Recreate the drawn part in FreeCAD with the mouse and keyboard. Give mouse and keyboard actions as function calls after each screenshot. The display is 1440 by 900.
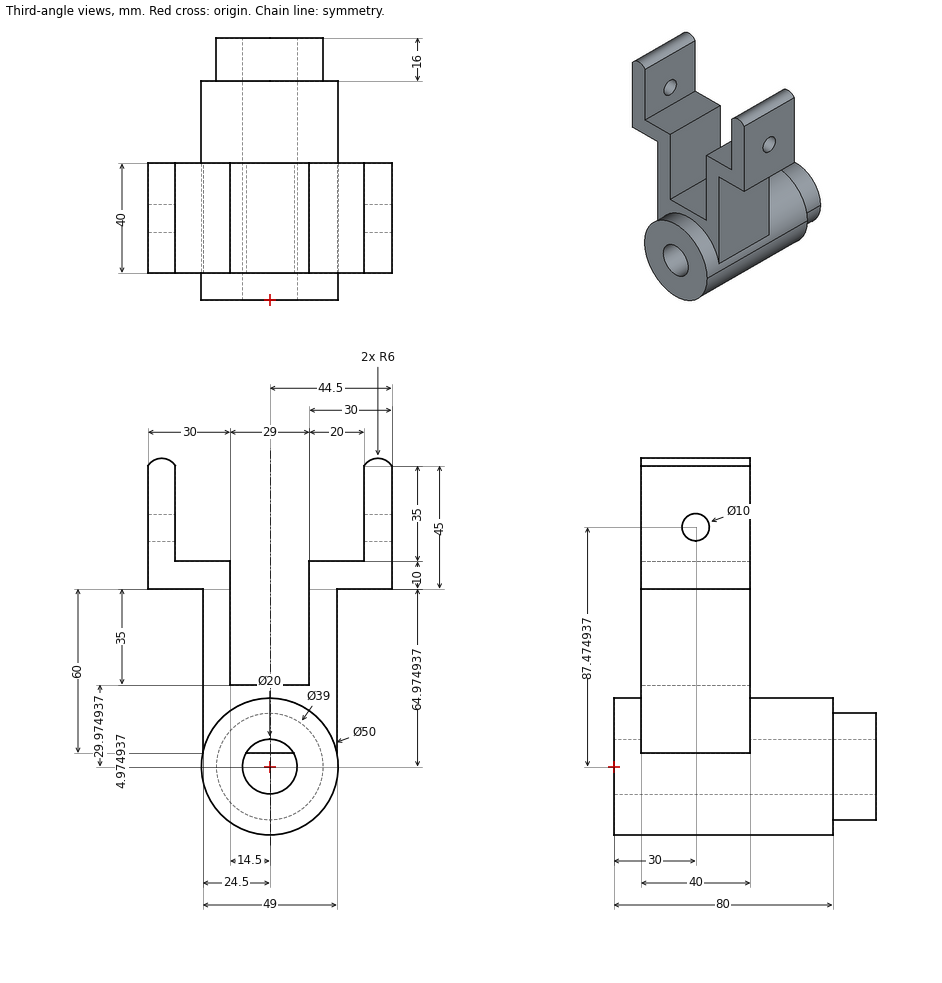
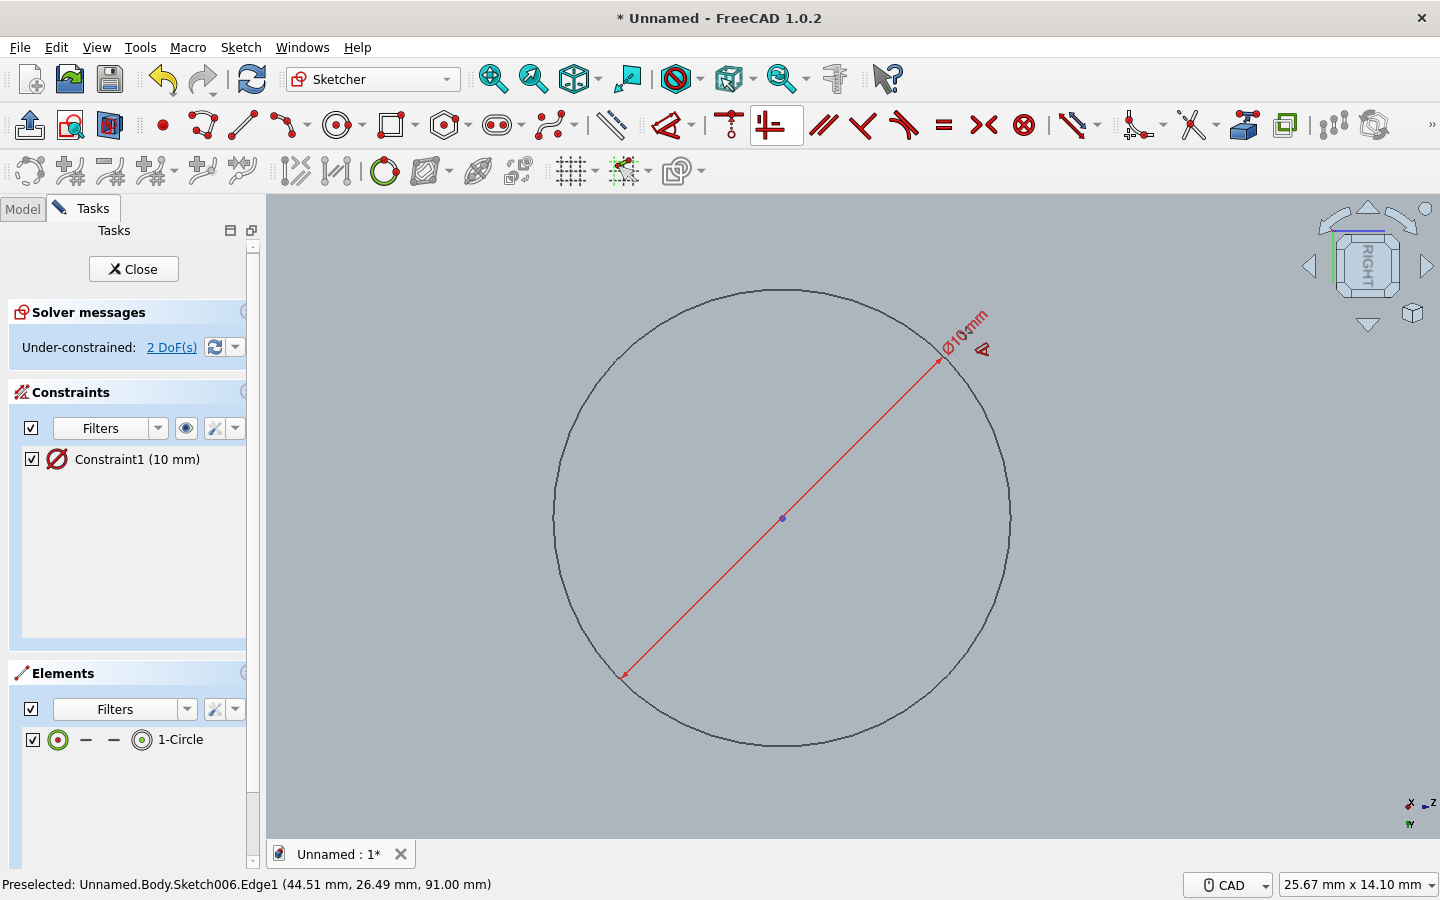
click(782, 518)
click(816, 370)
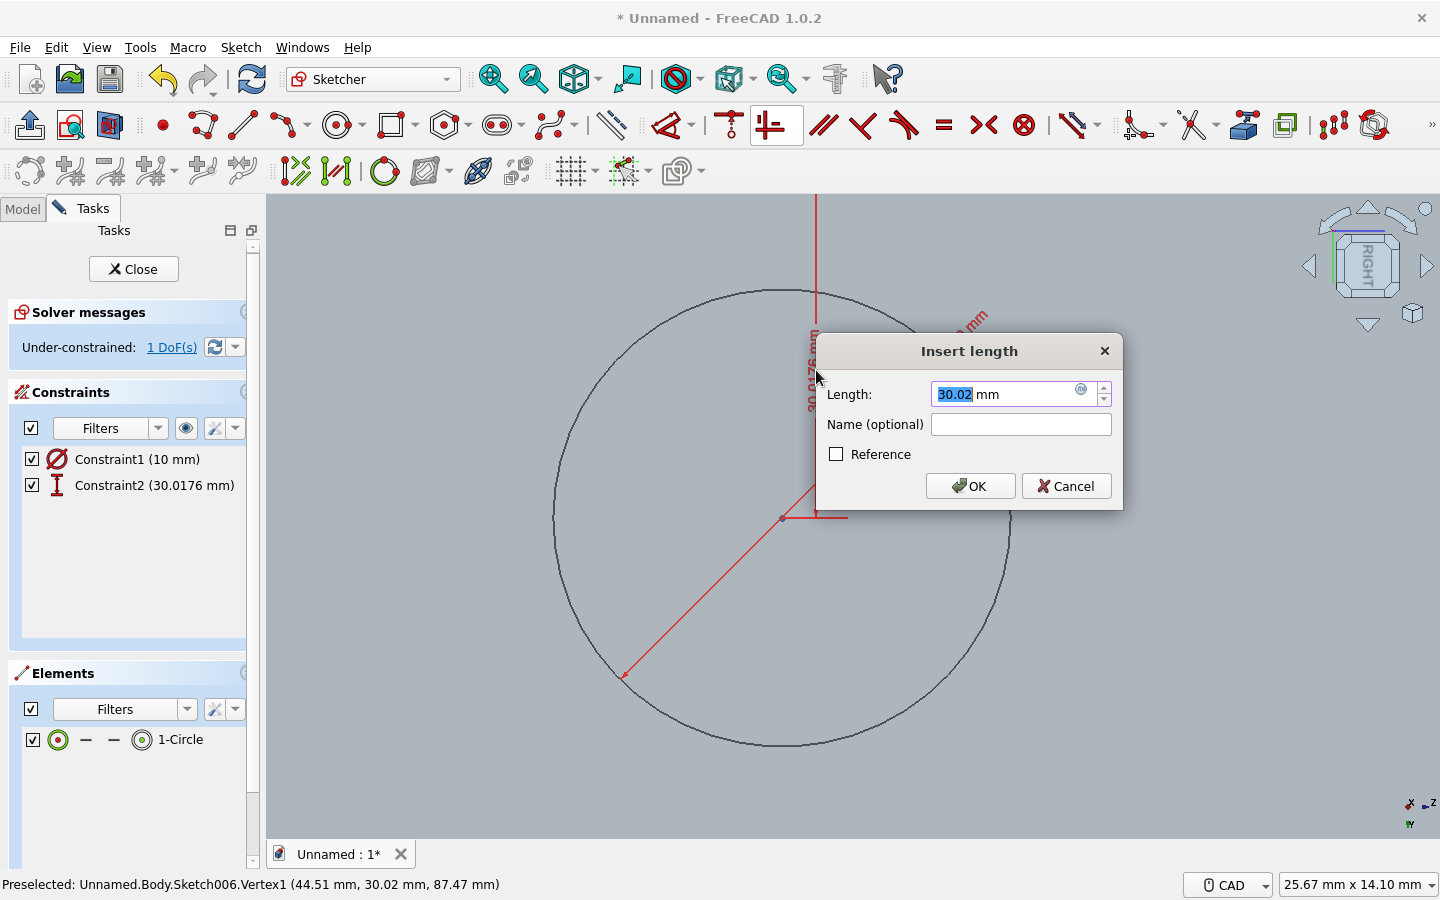
text(30)
key(Return)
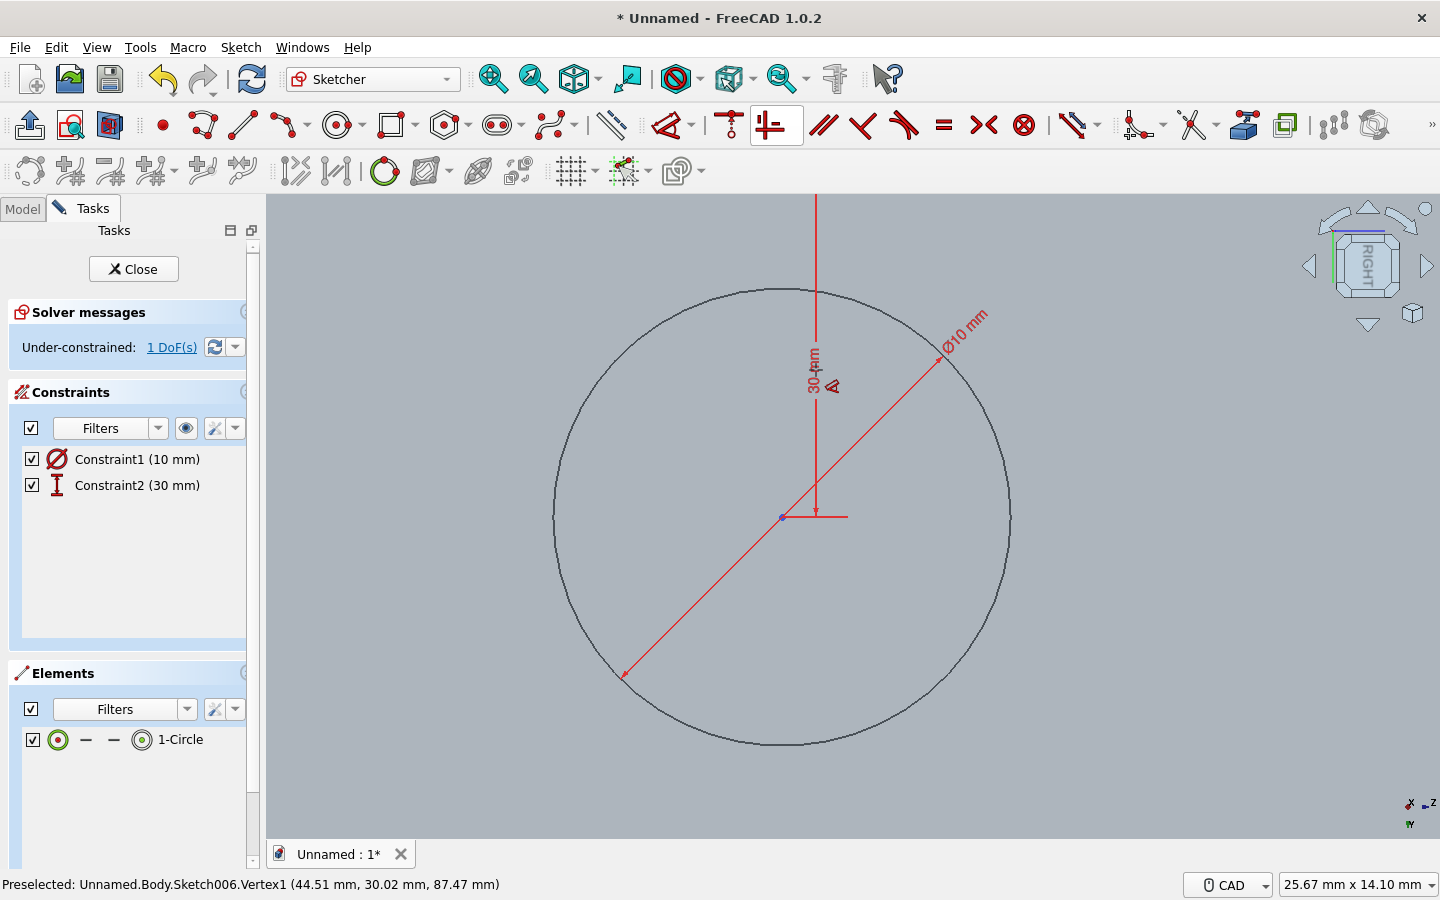
click(782, 517)
click(538, 551)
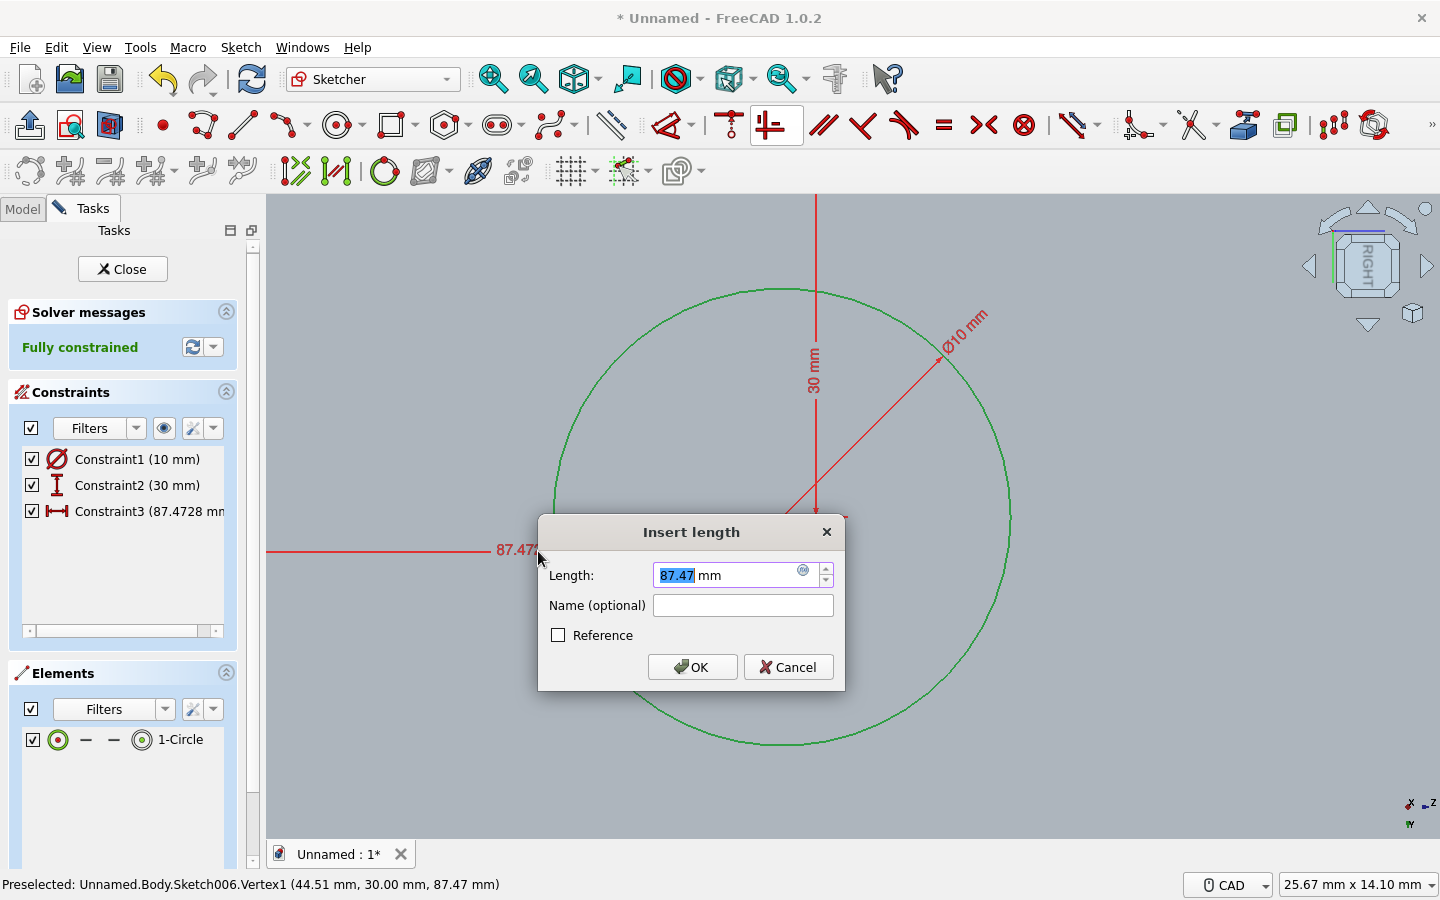
text(87.474937)
key(Return)
key(Escape)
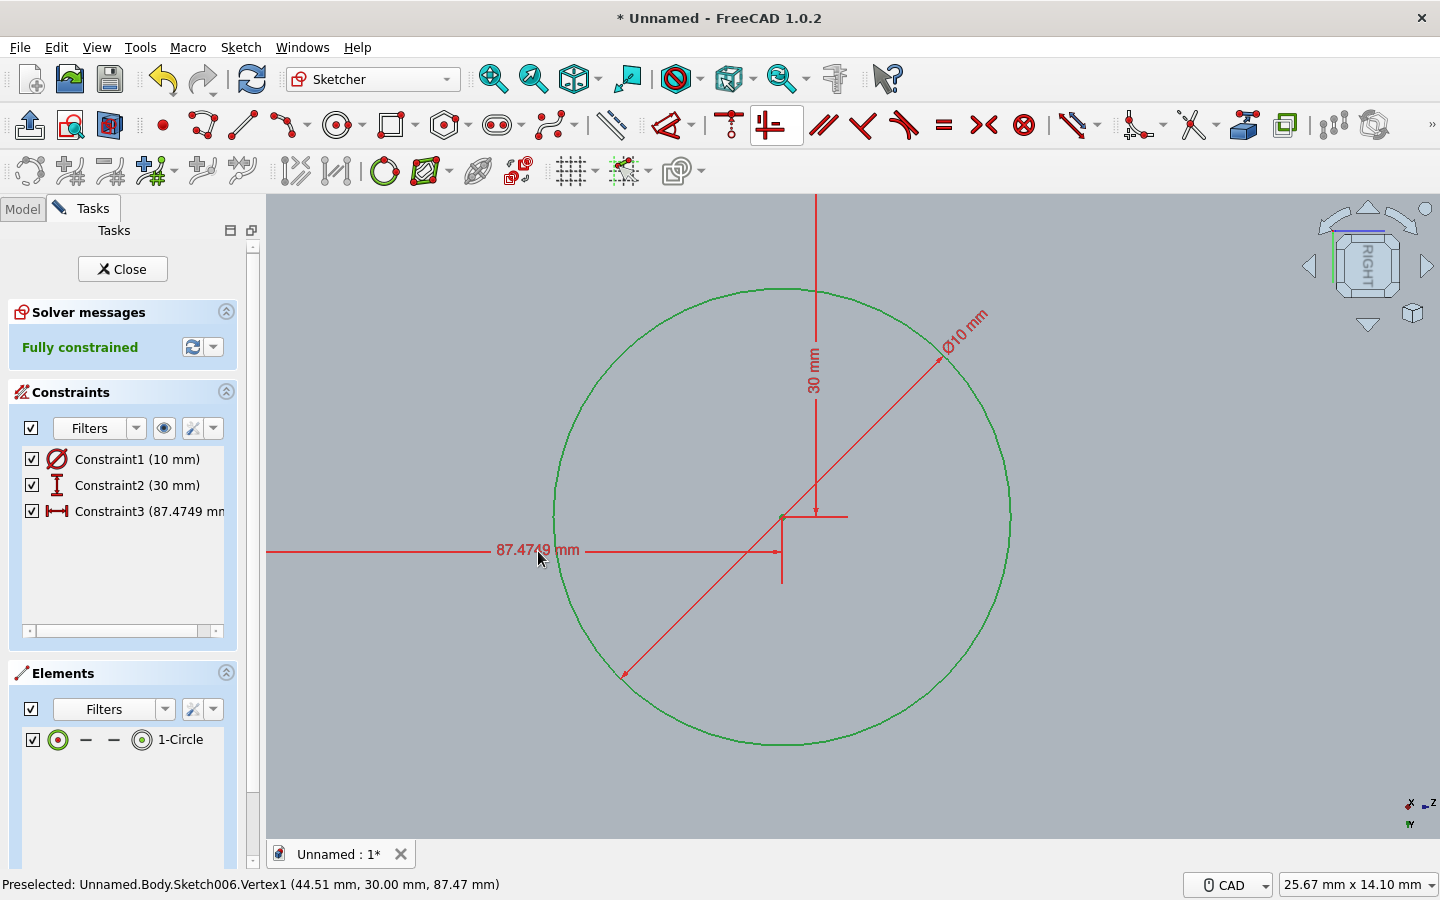
click(123, 269)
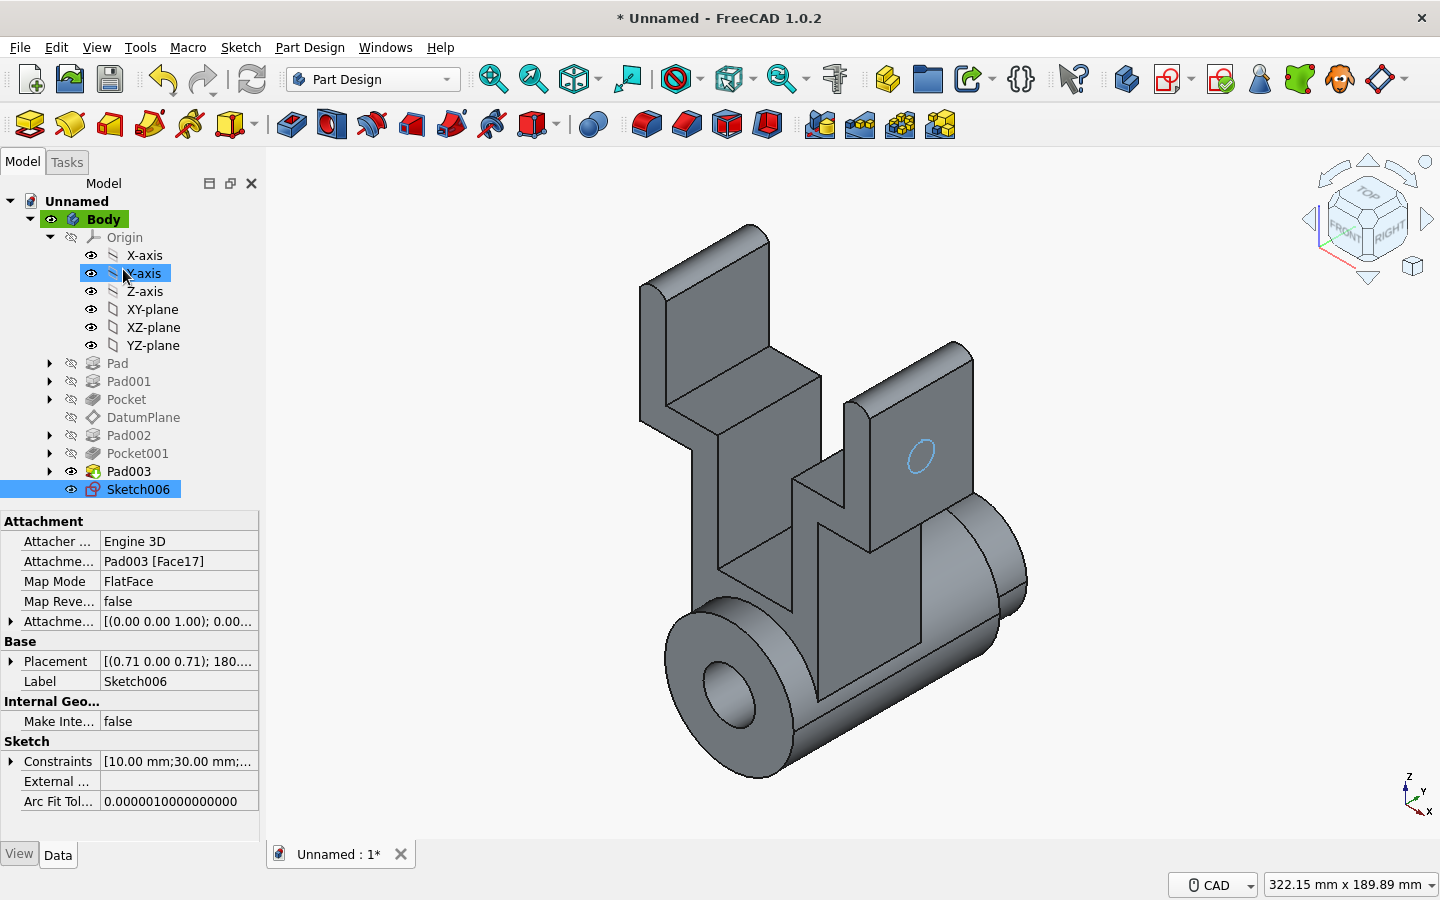
click(292, 124)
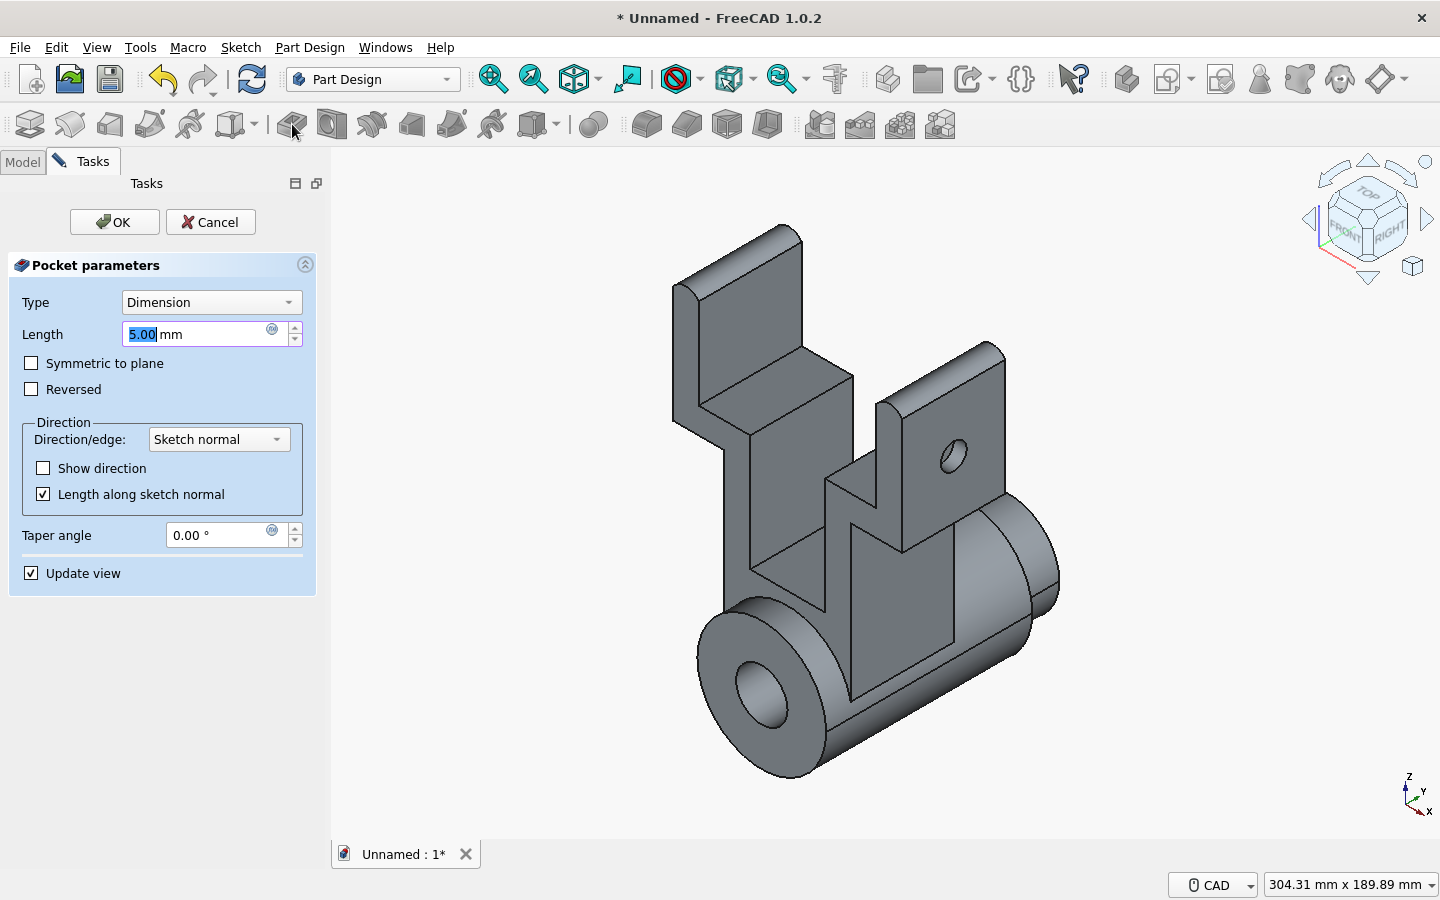
click(212, 302)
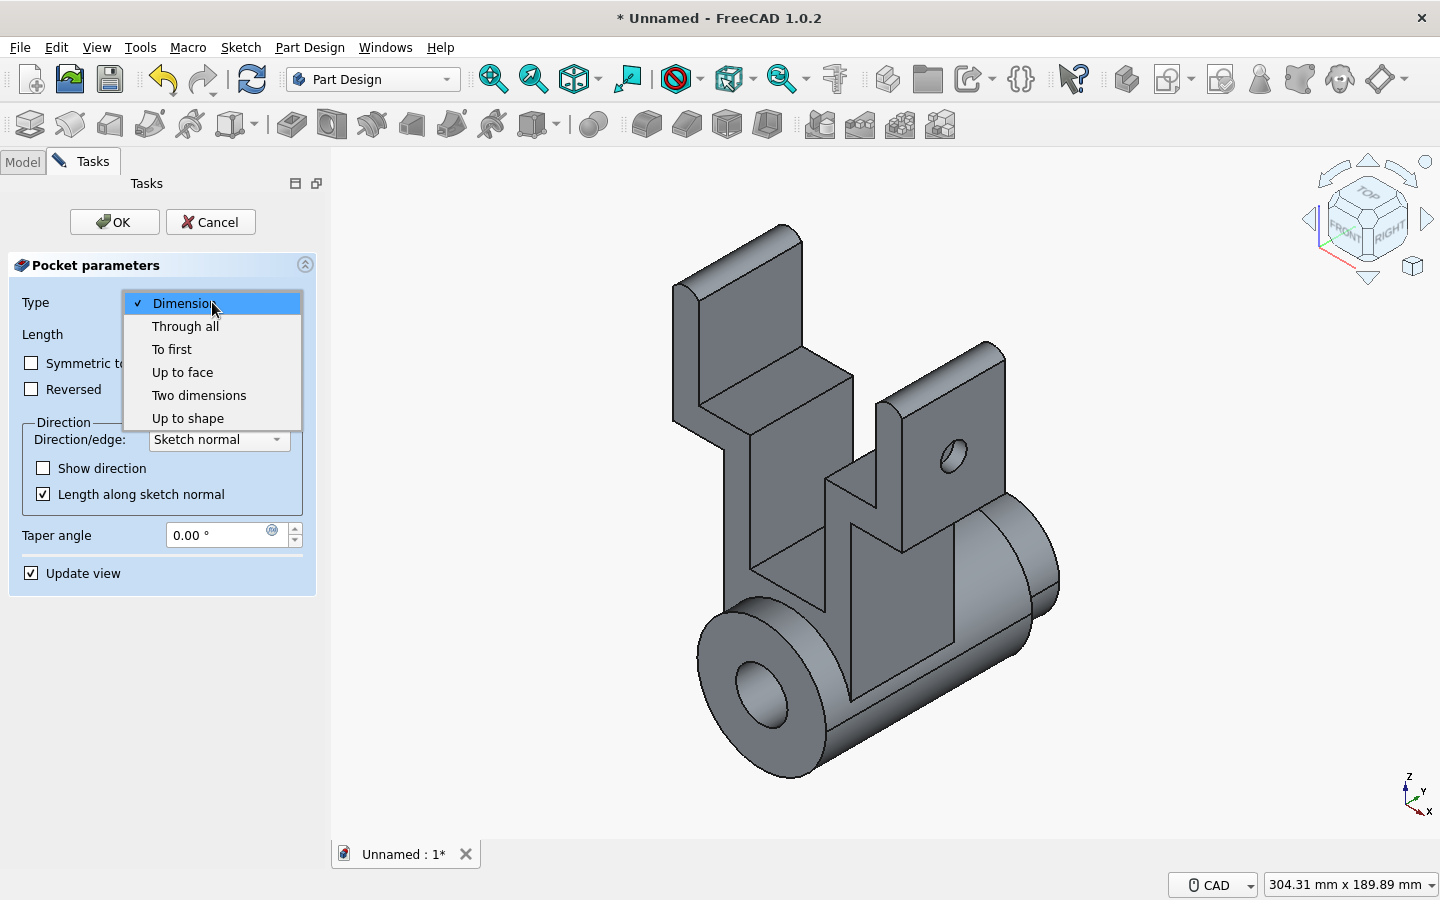
click(212, 326)